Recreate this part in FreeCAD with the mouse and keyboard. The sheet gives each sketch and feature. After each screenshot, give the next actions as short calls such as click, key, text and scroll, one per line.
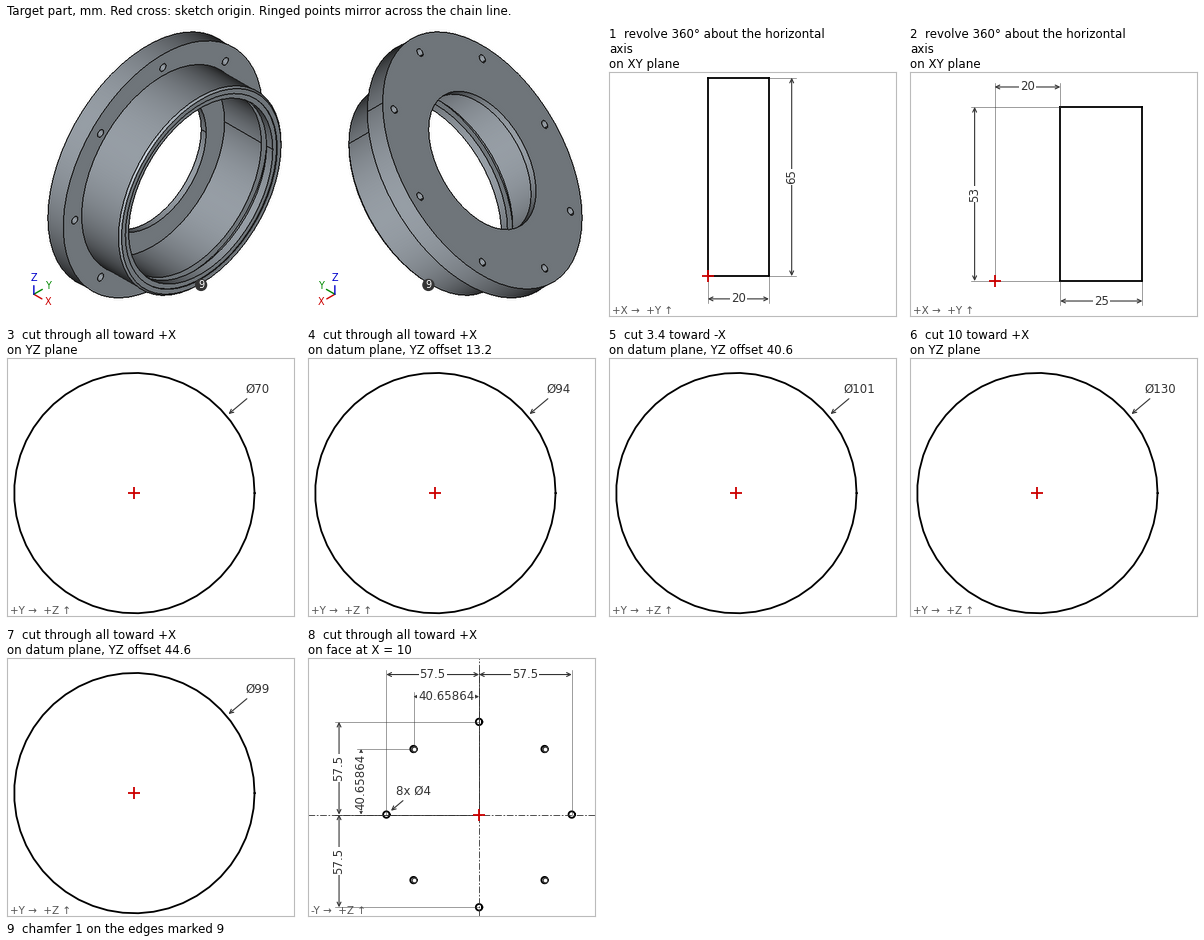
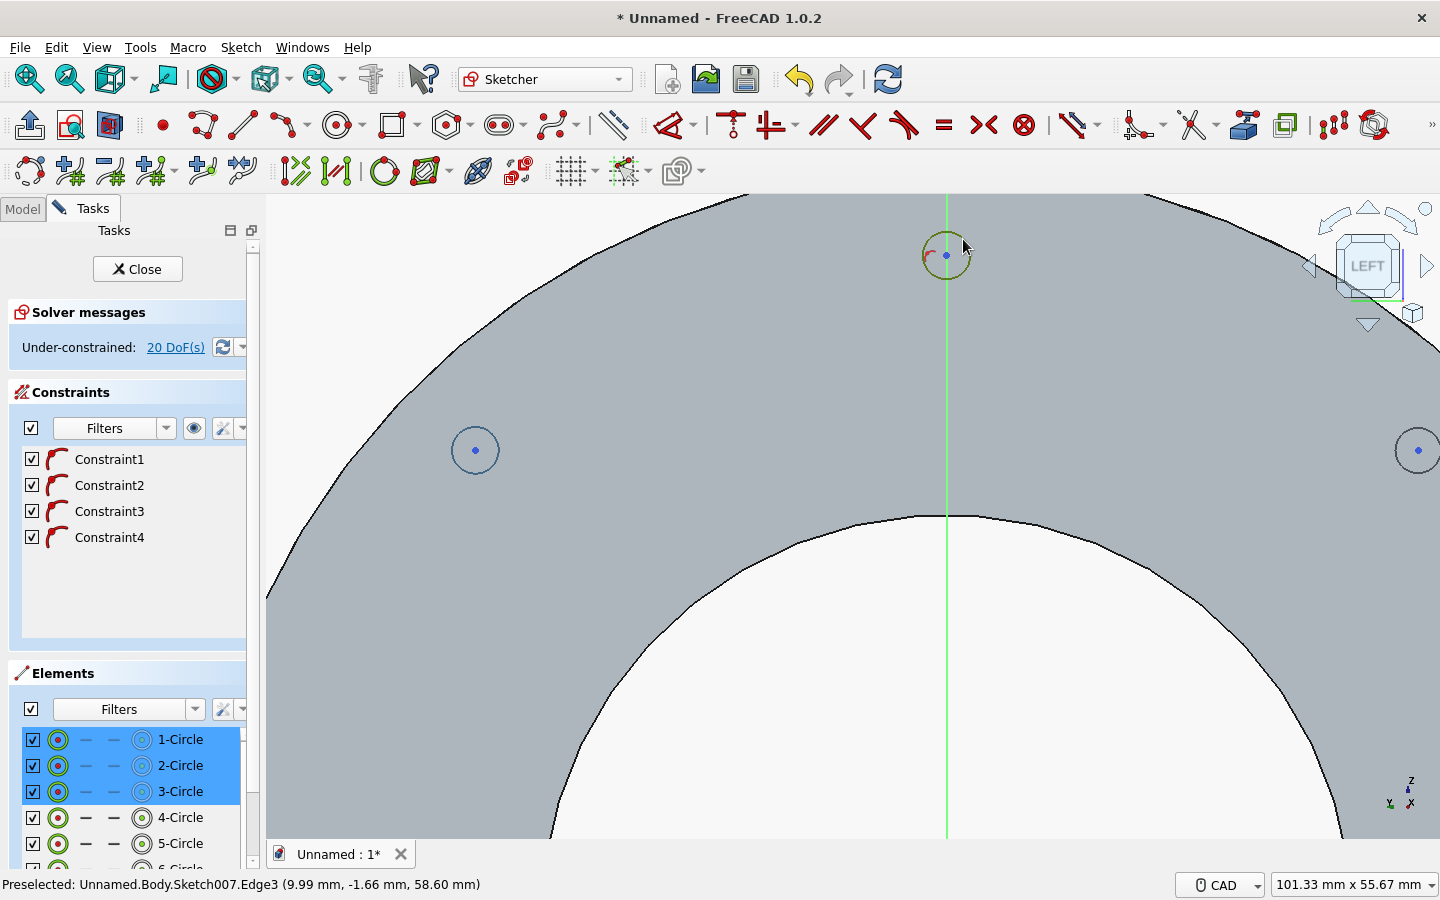
scroll(715, 342, down, 6)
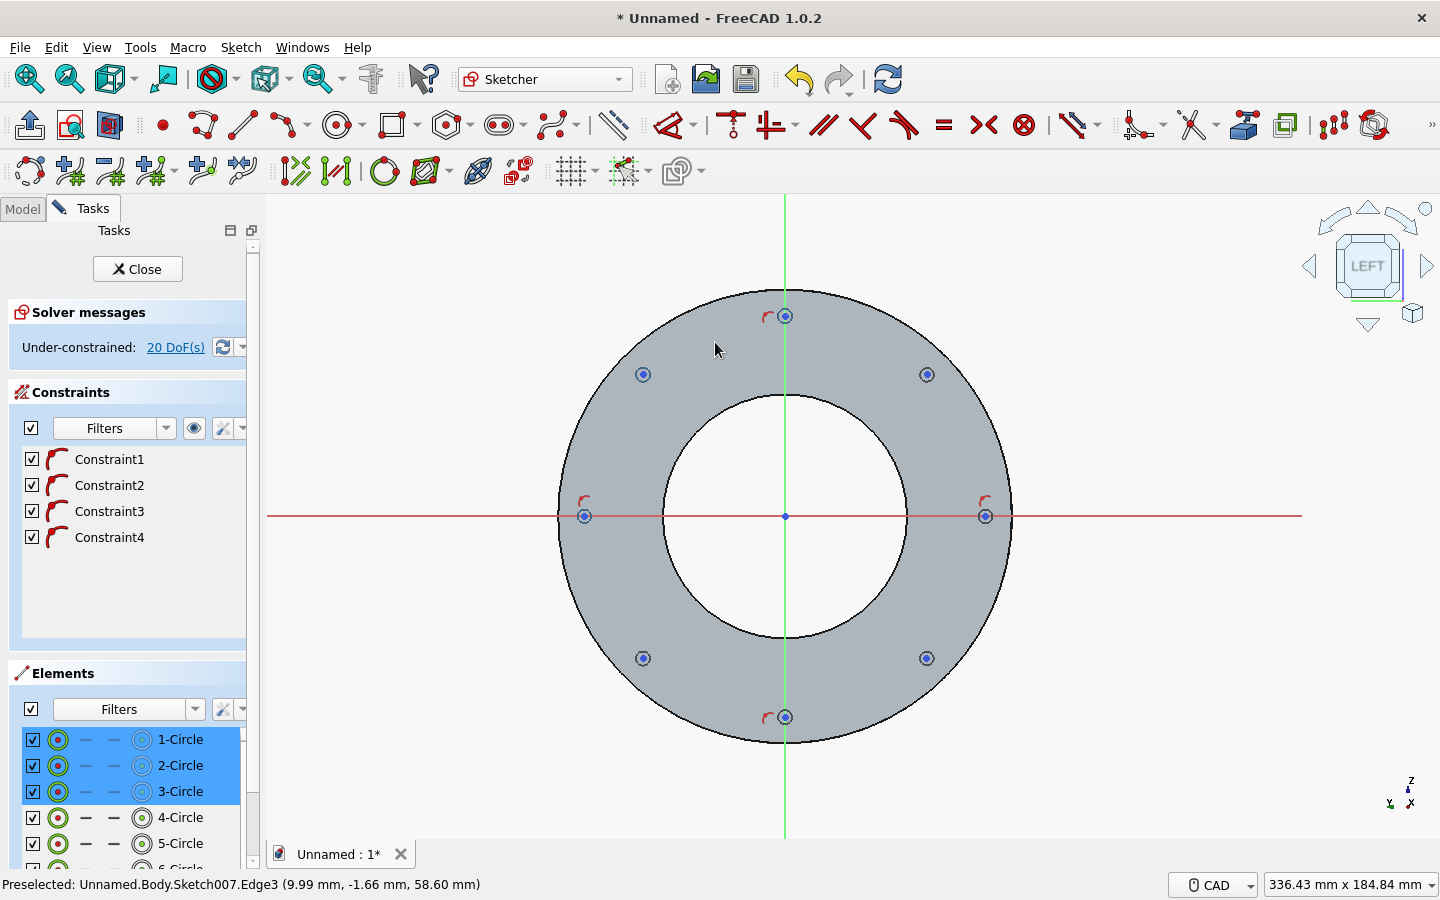
scroll(932, 370, up, 4)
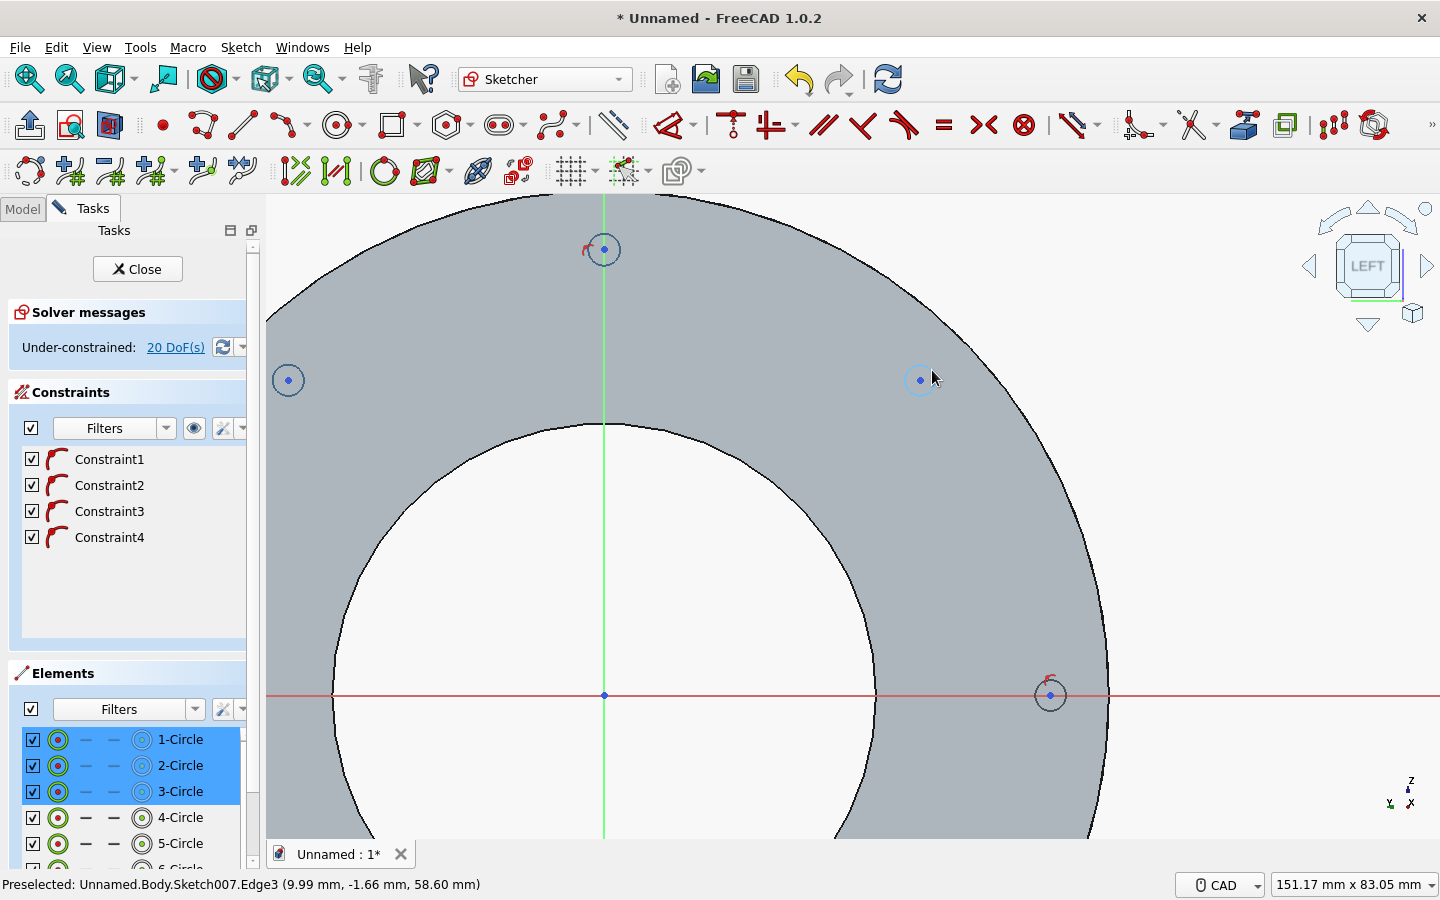
click(931, 370)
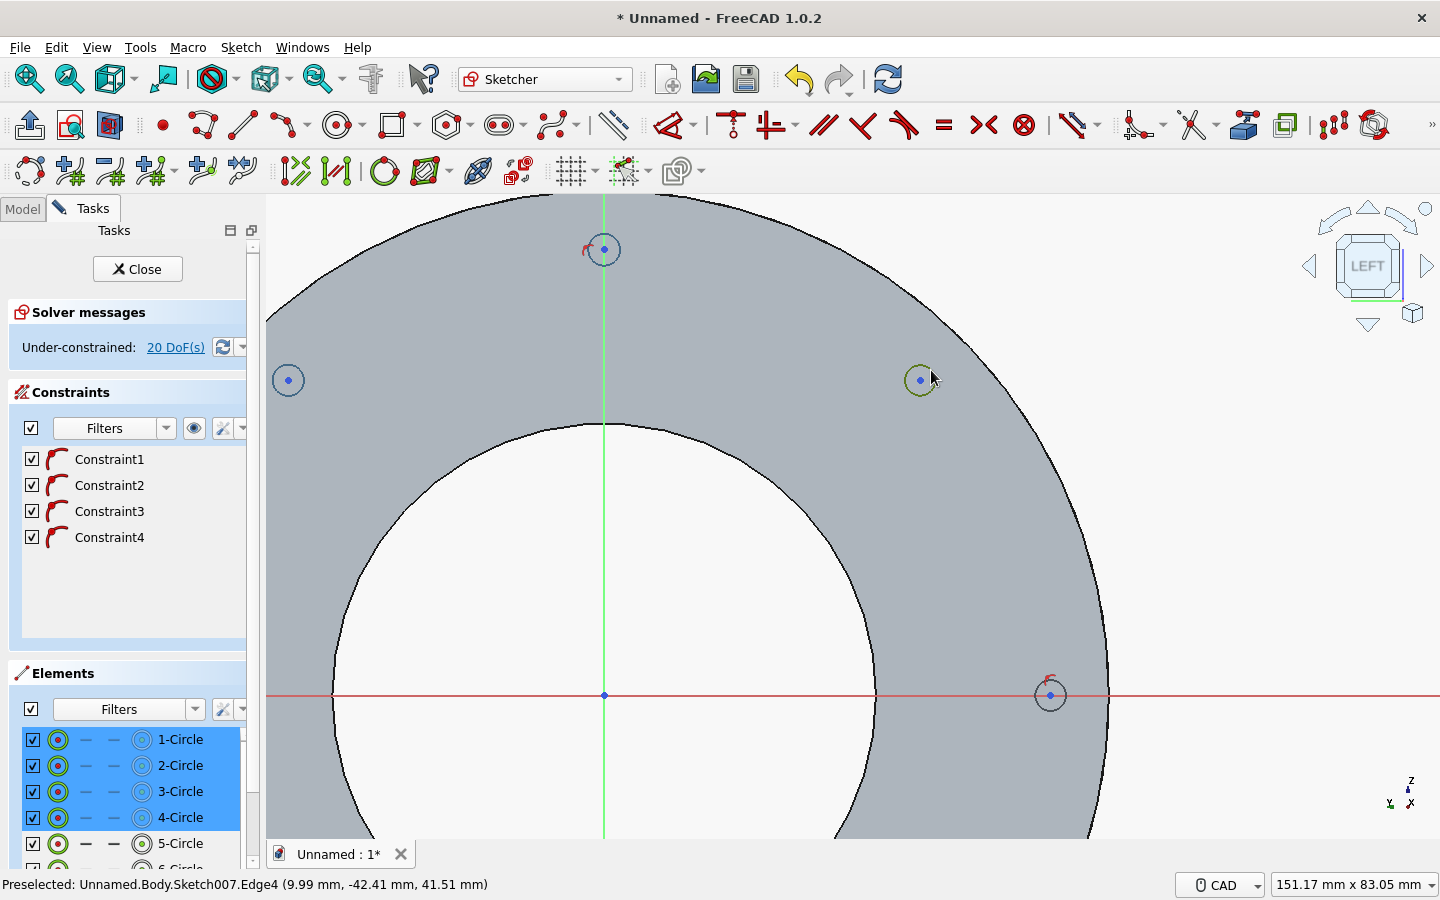
scroll(1061, 685, up, 2)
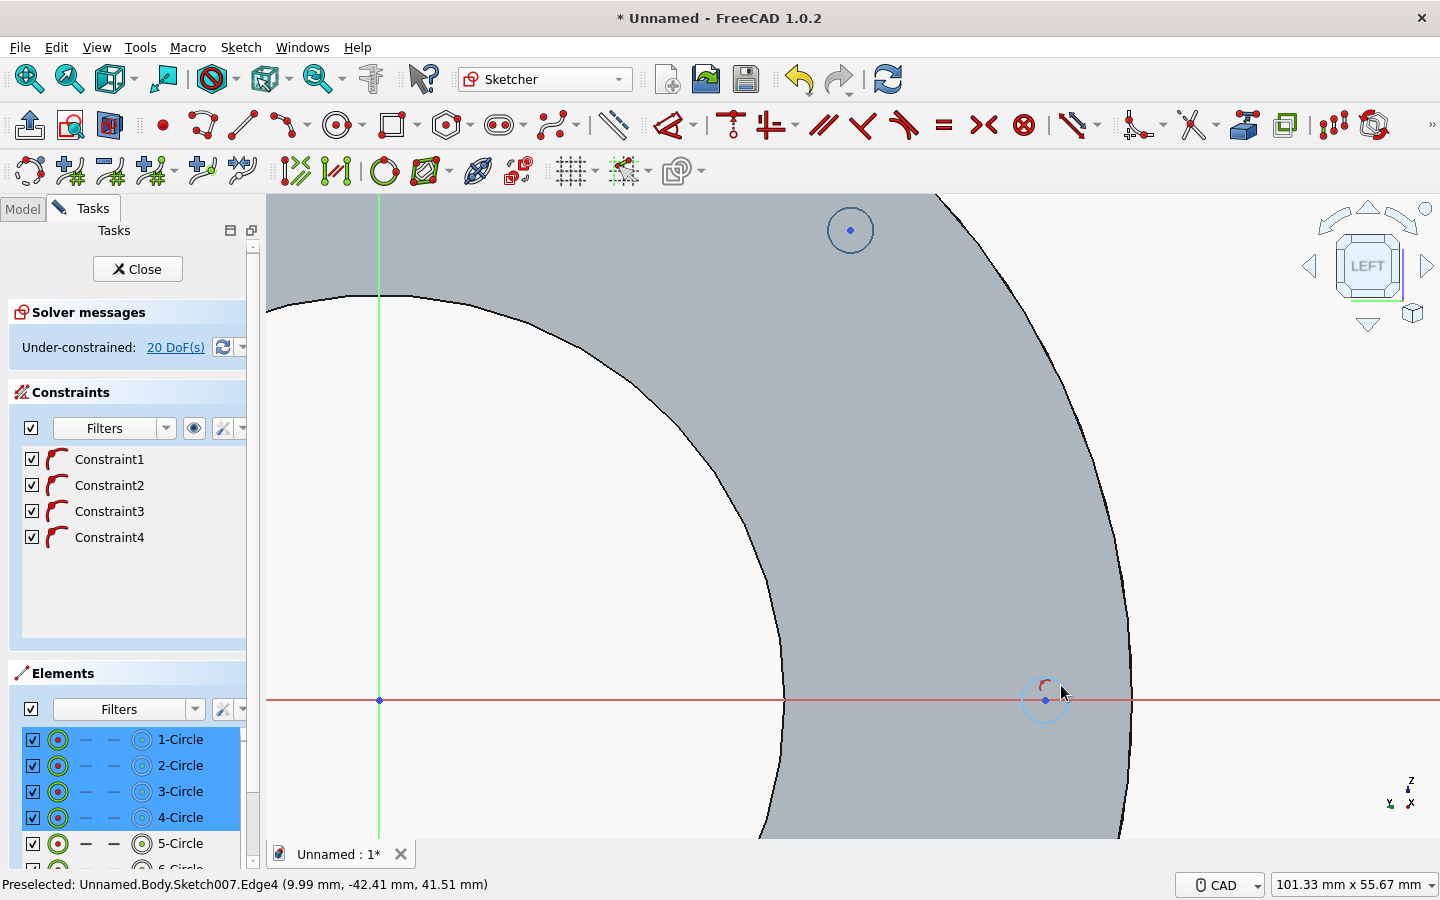
click(1061, 684)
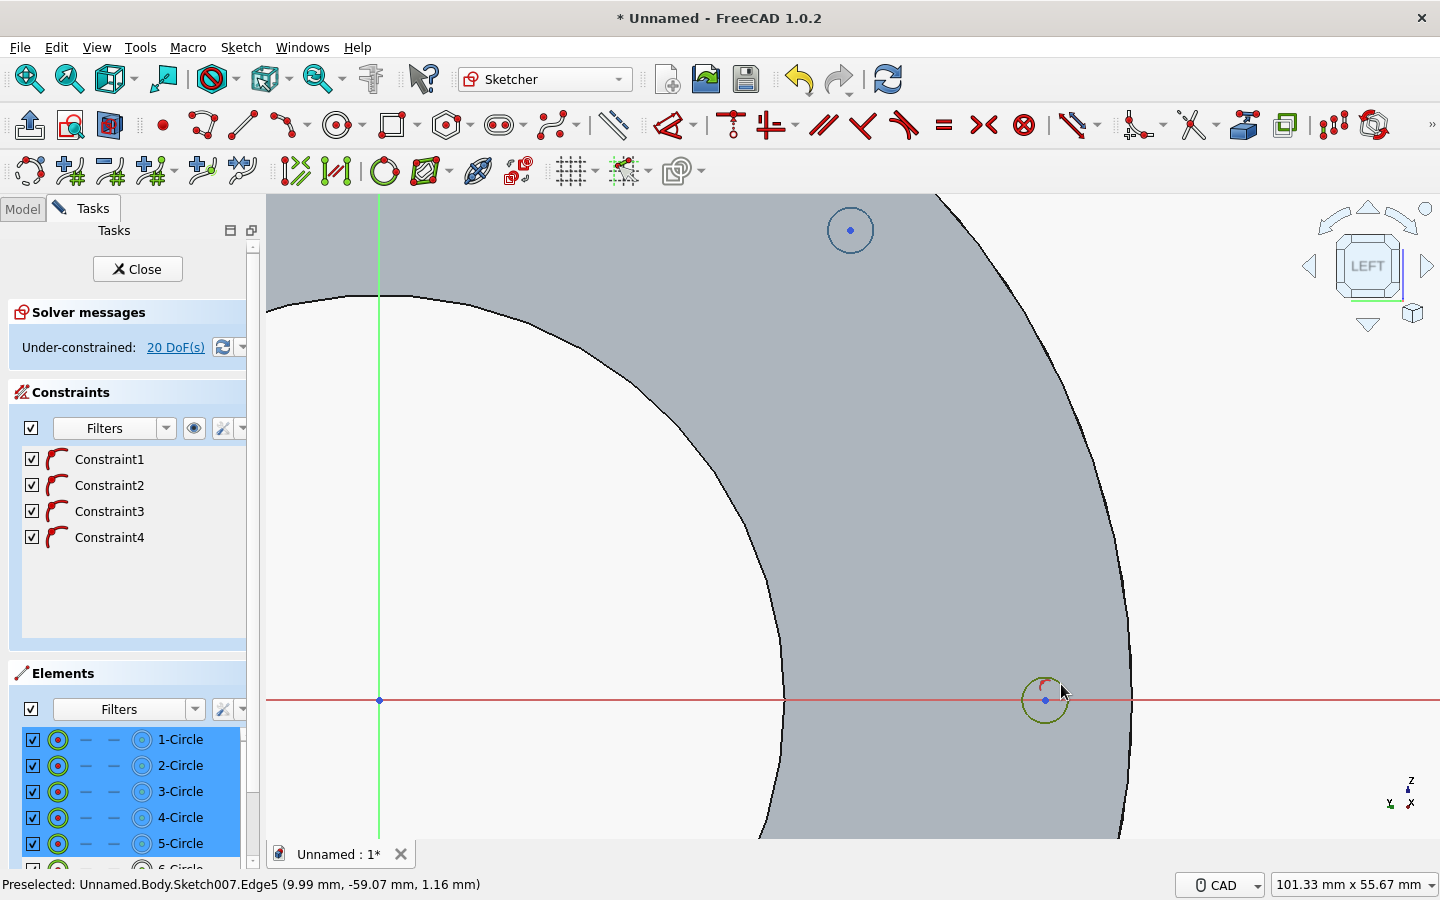
scroll(959, 437, down, 6)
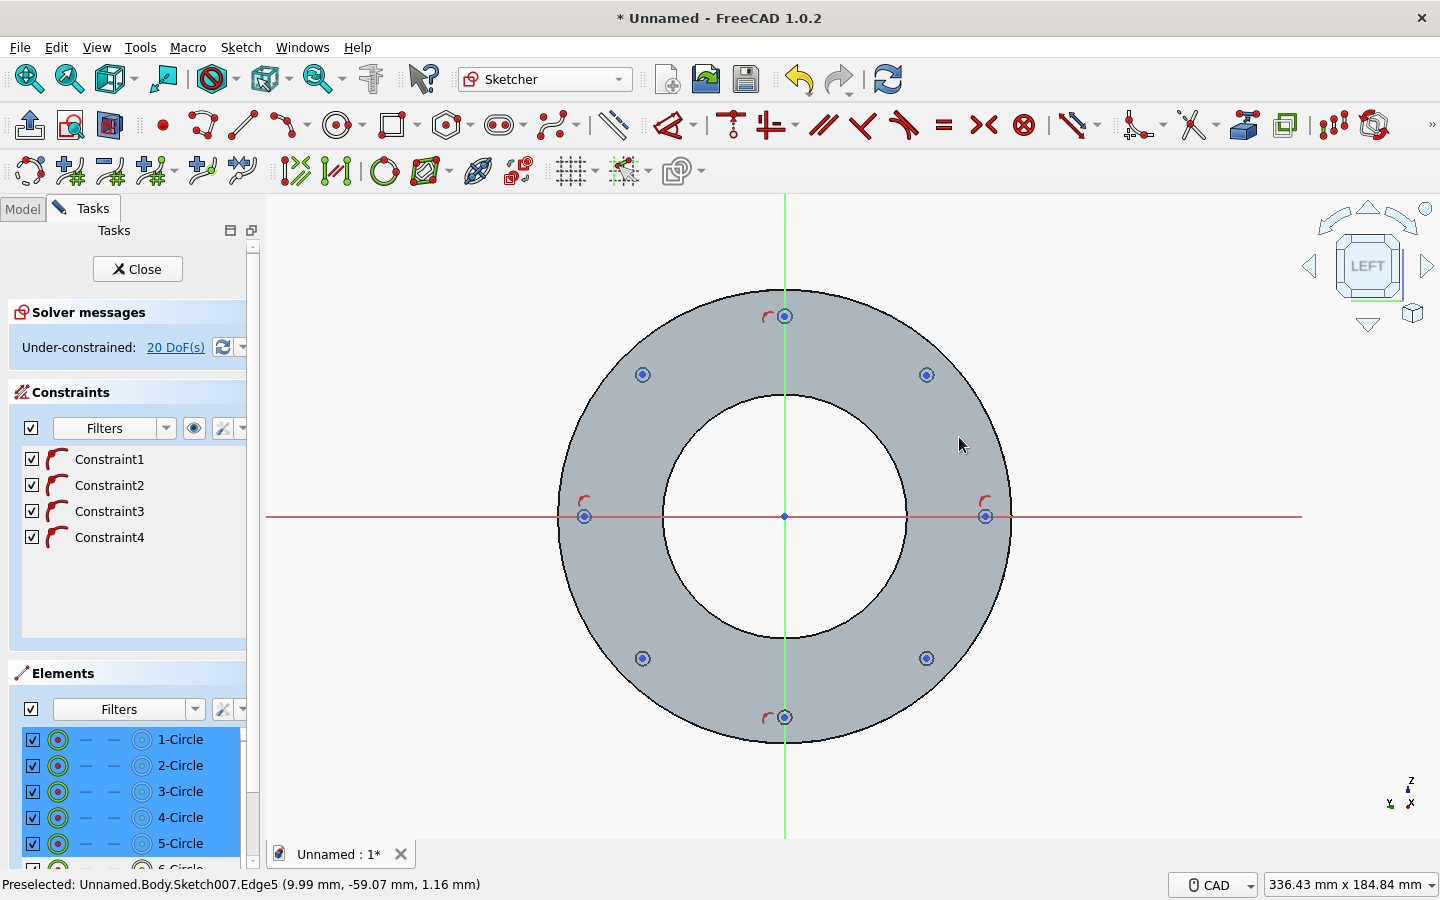
scroll(932, 654, up, 4)